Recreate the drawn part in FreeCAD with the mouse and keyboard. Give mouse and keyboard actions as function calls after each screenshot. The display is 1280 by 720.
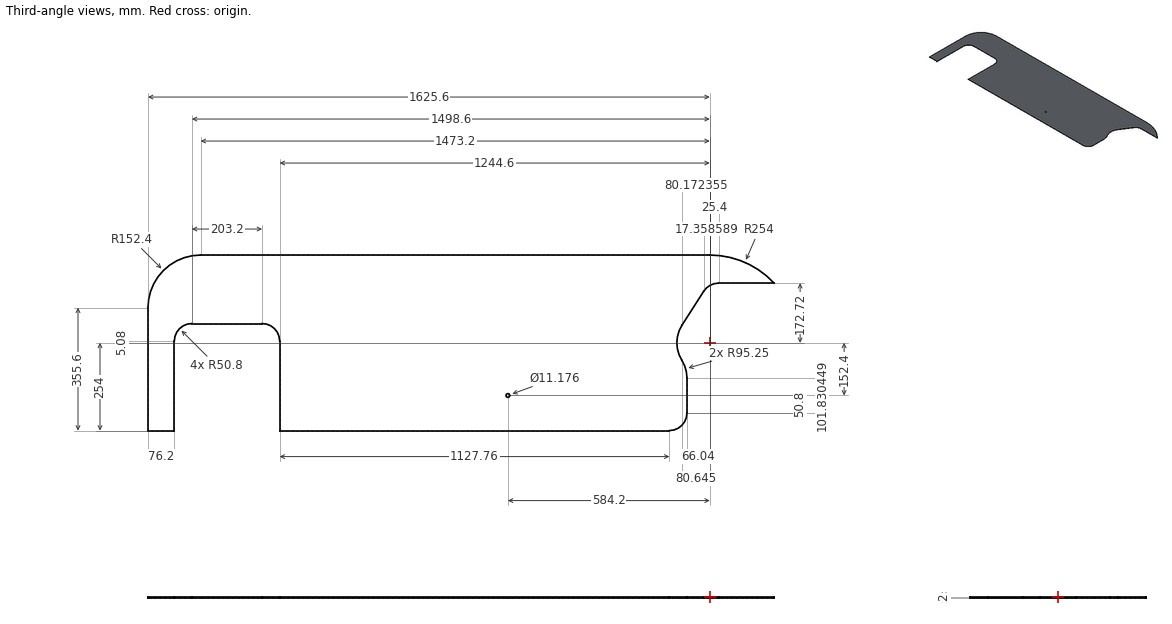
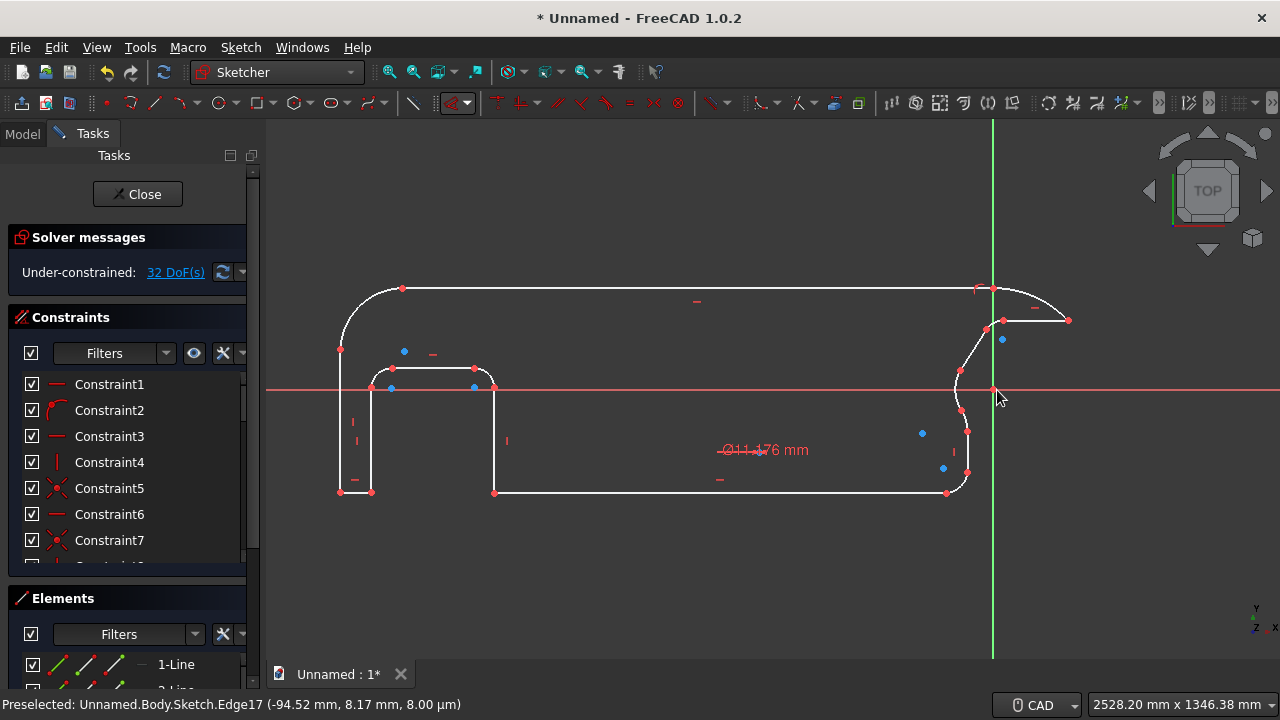
scroll(383, 370, up, 2)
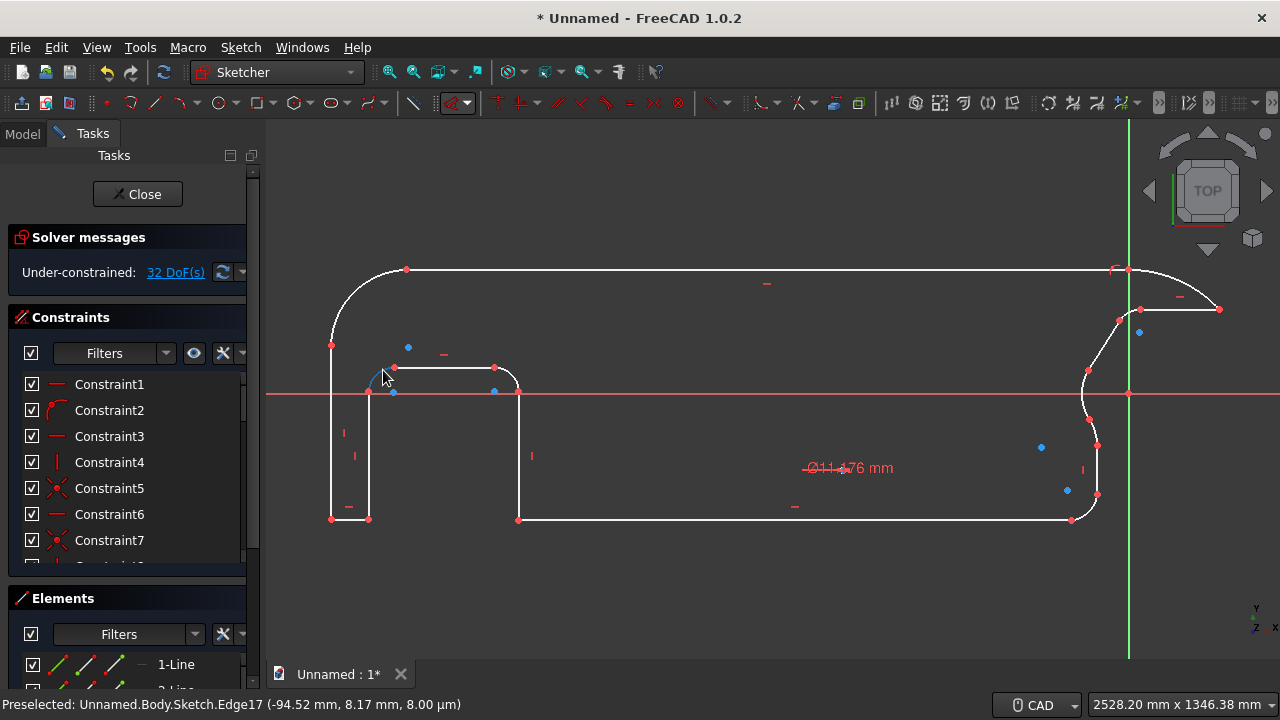
click(383, 370)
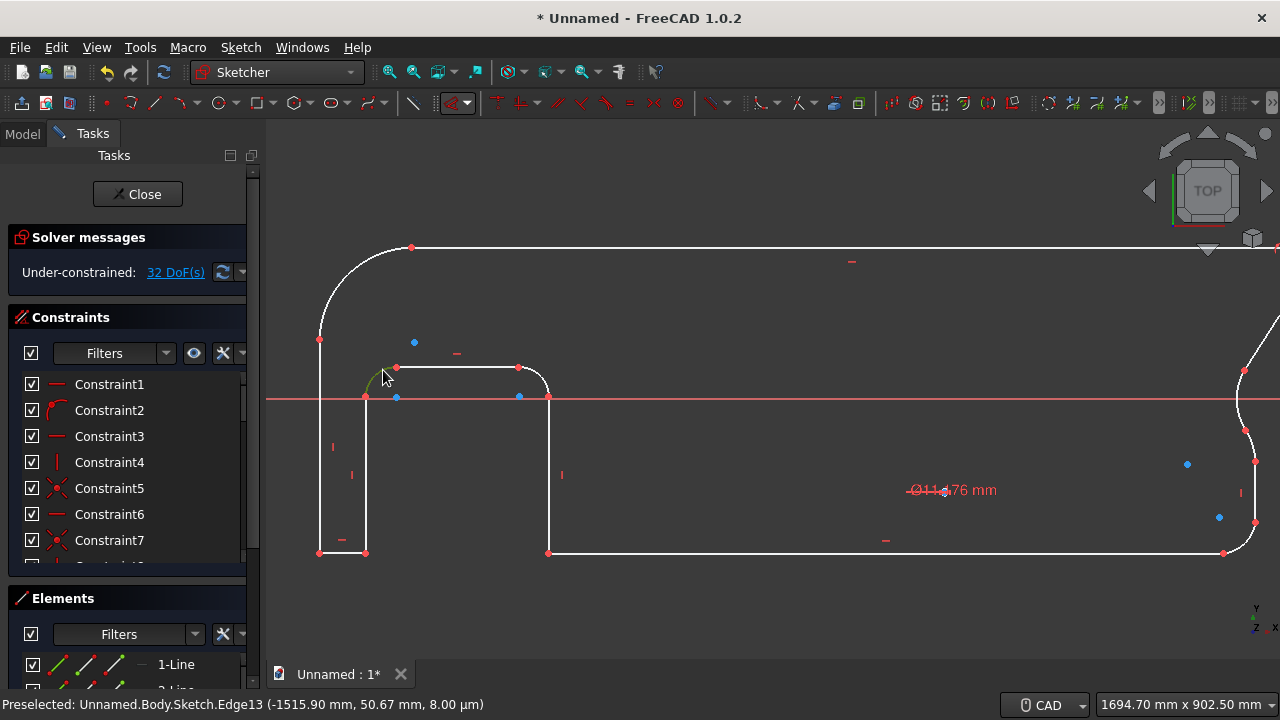
click(545, 383)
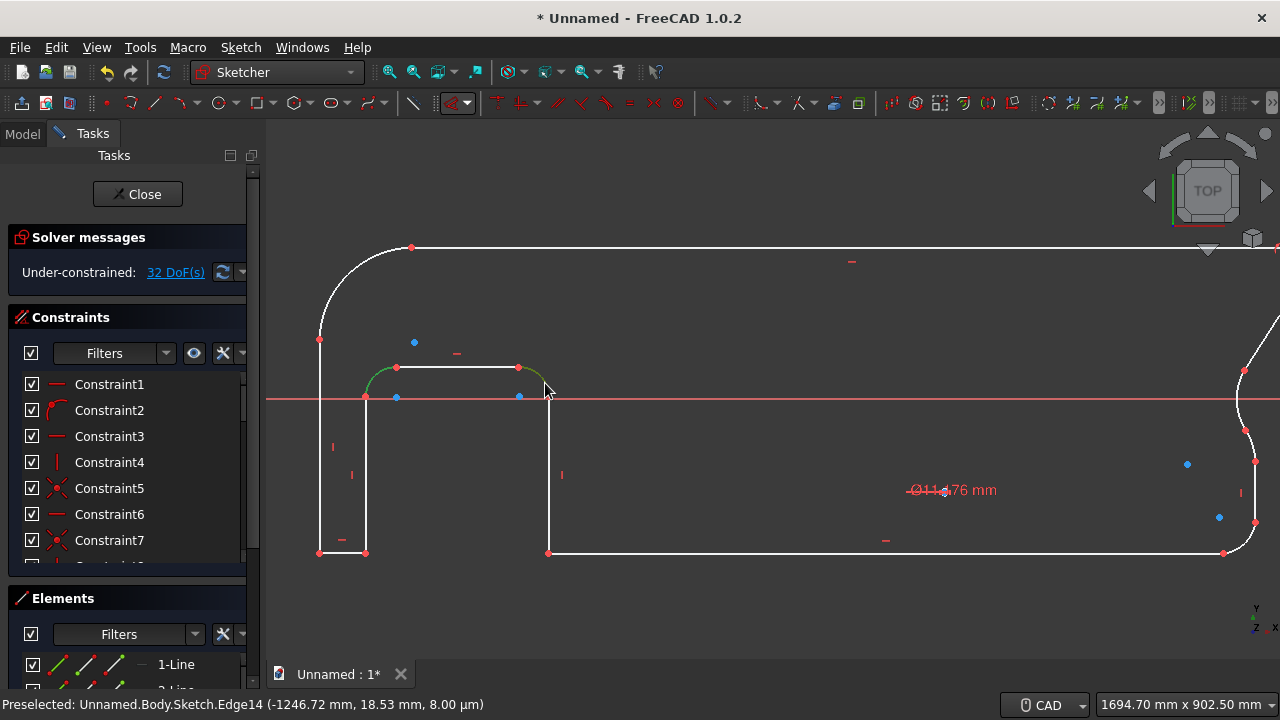
scroll(512, 377, down, 3)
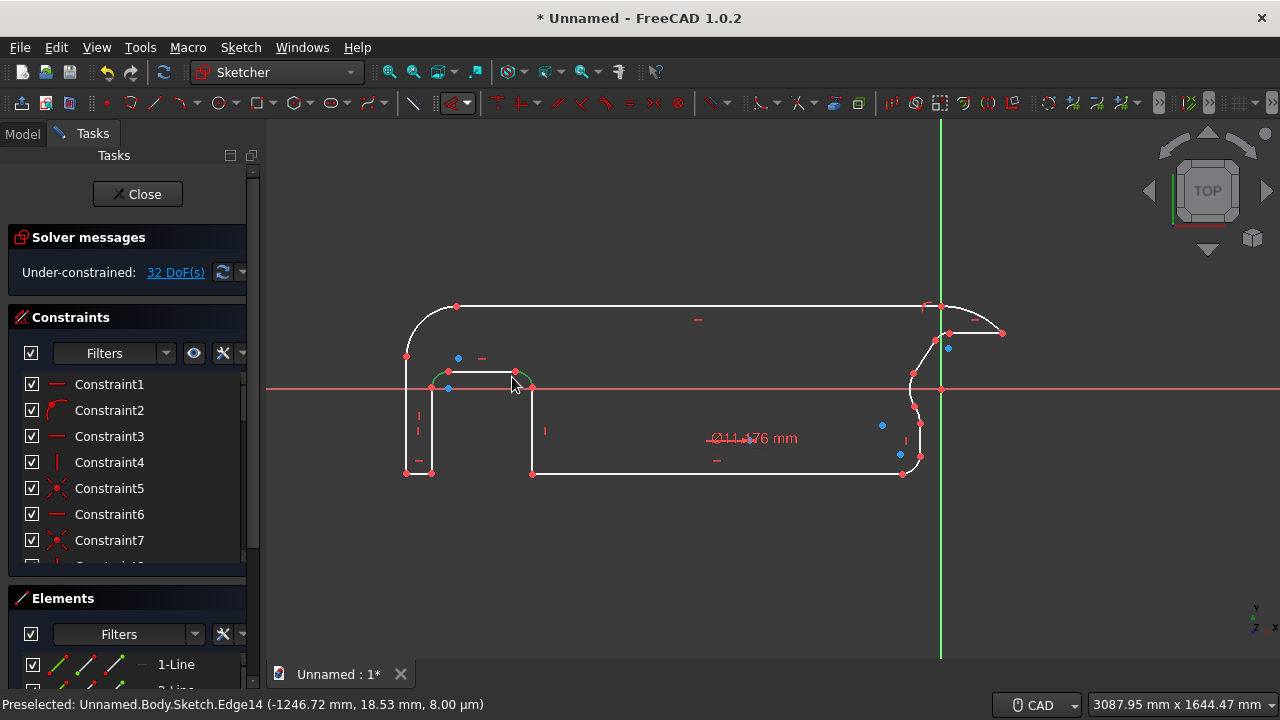
scroll(910, 472, up, 3)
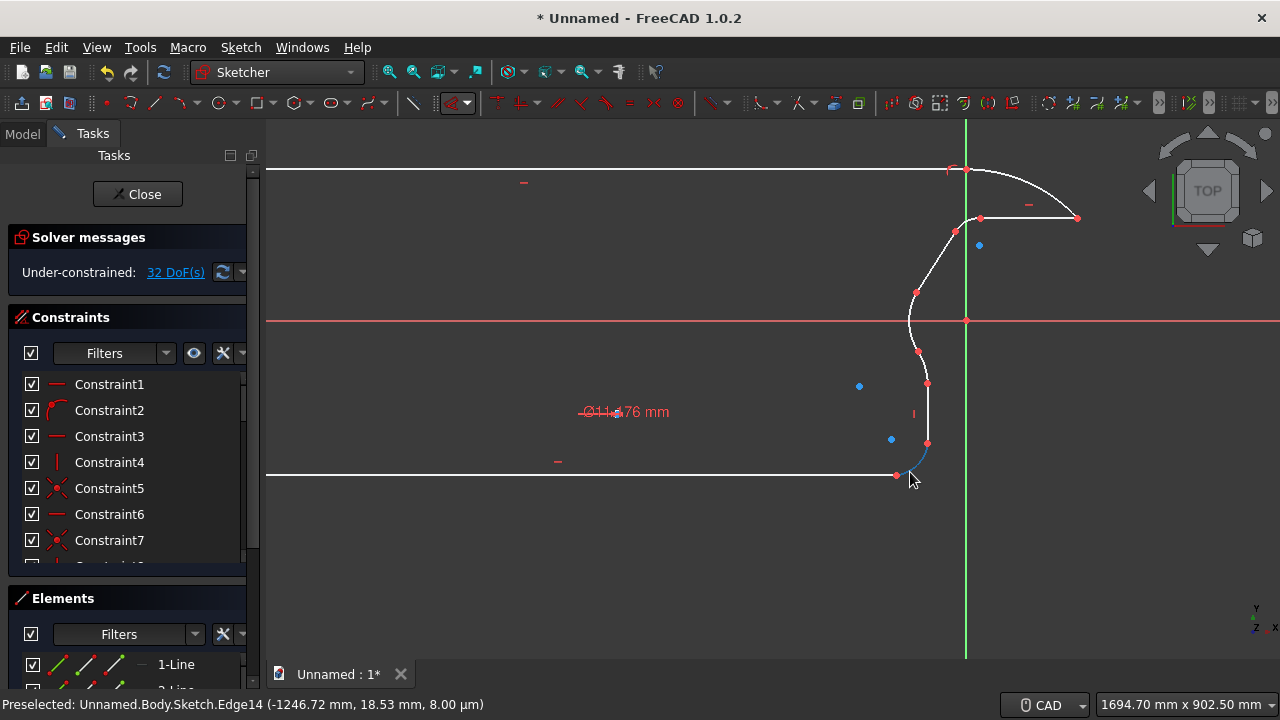
click(910, 471)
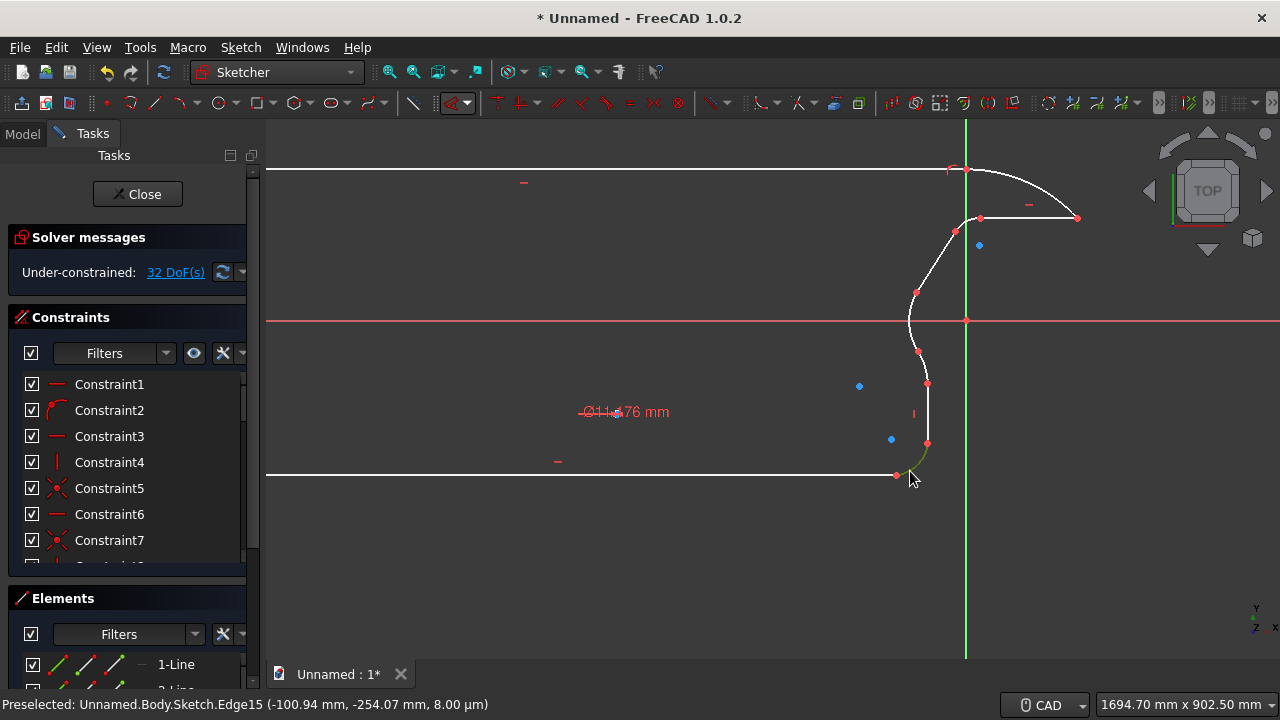
click(966, 221)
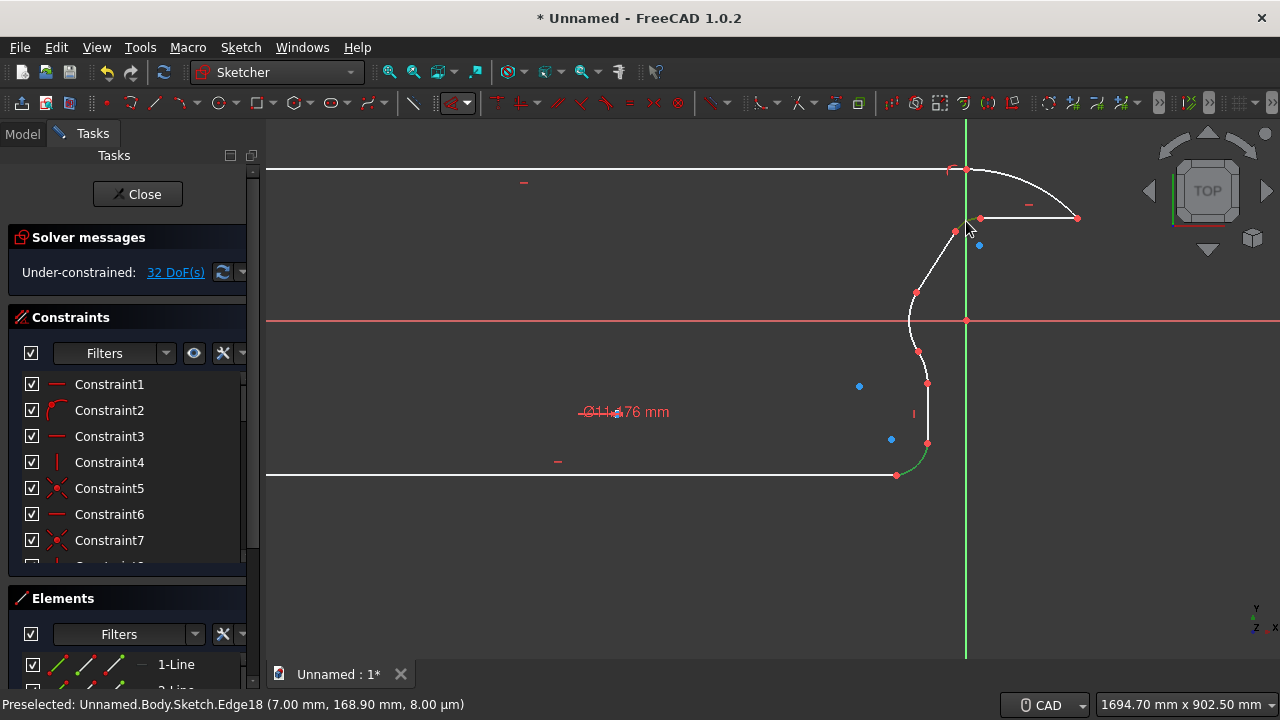
click(630, 104)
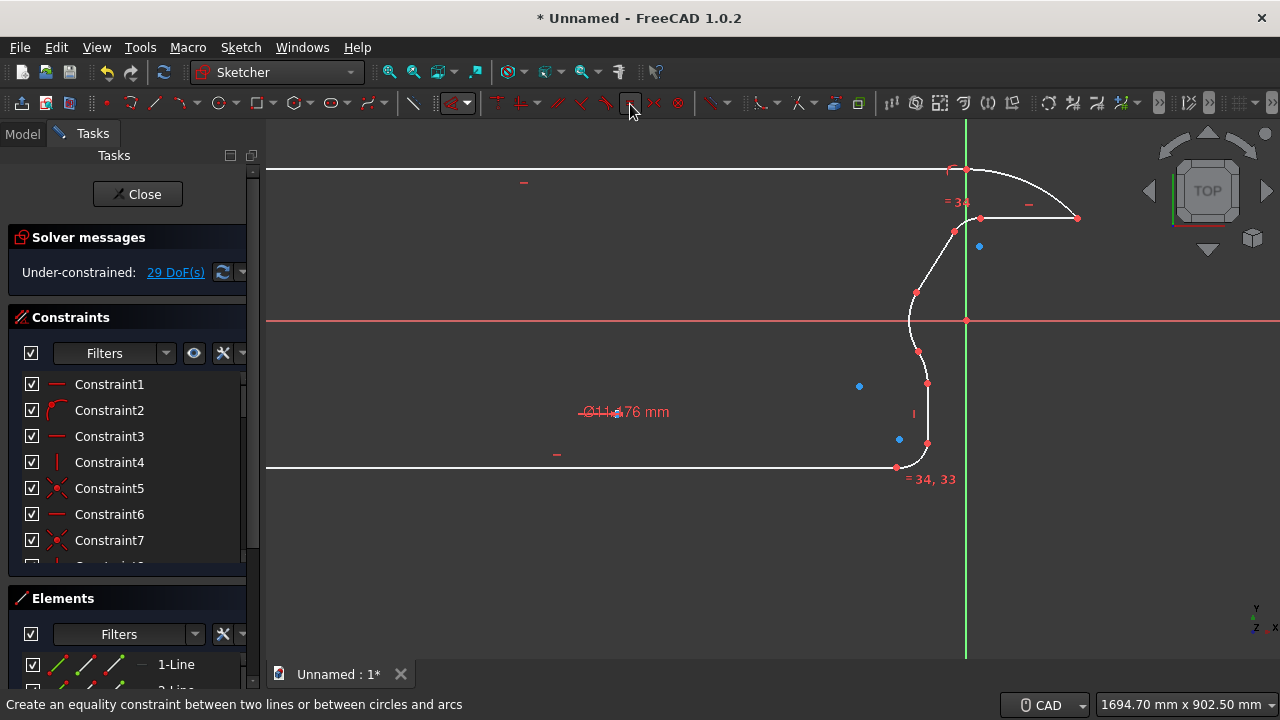
scroll(927, 374, up, 2)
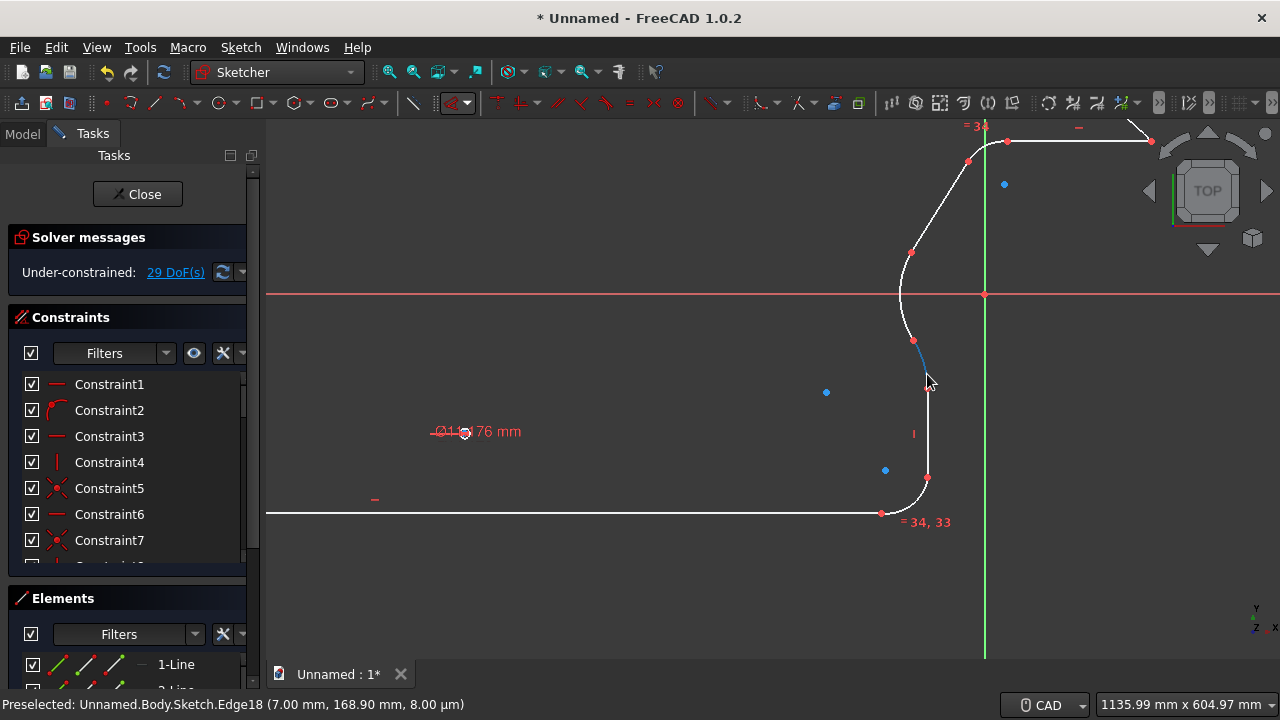
click(926, 373)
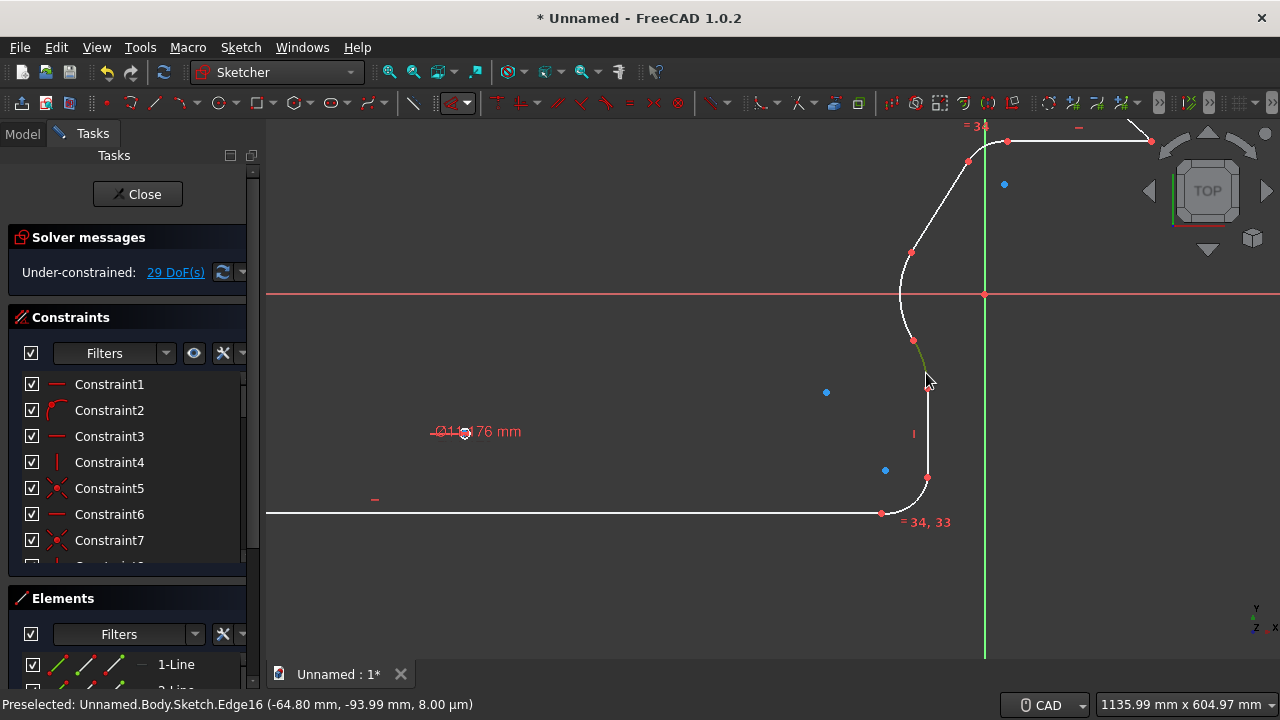
click(902, 278)